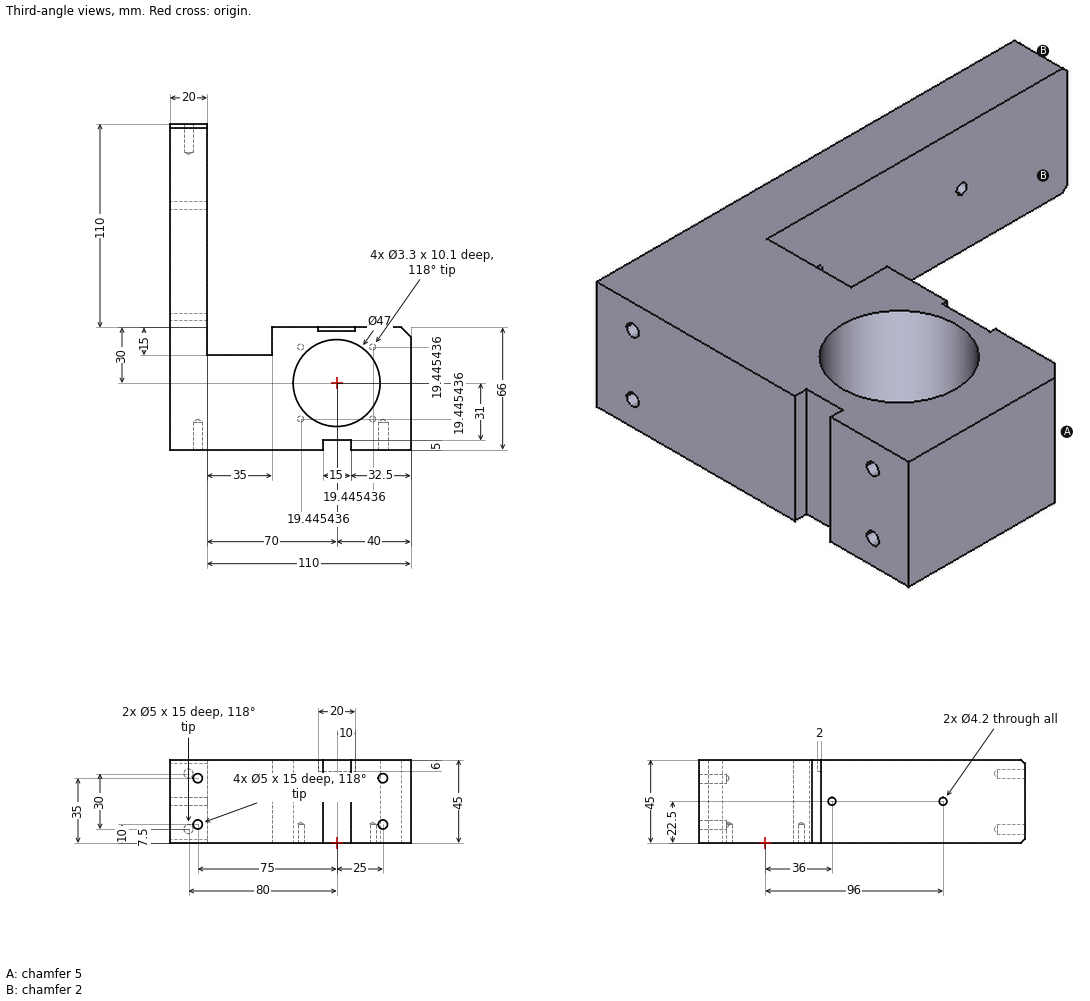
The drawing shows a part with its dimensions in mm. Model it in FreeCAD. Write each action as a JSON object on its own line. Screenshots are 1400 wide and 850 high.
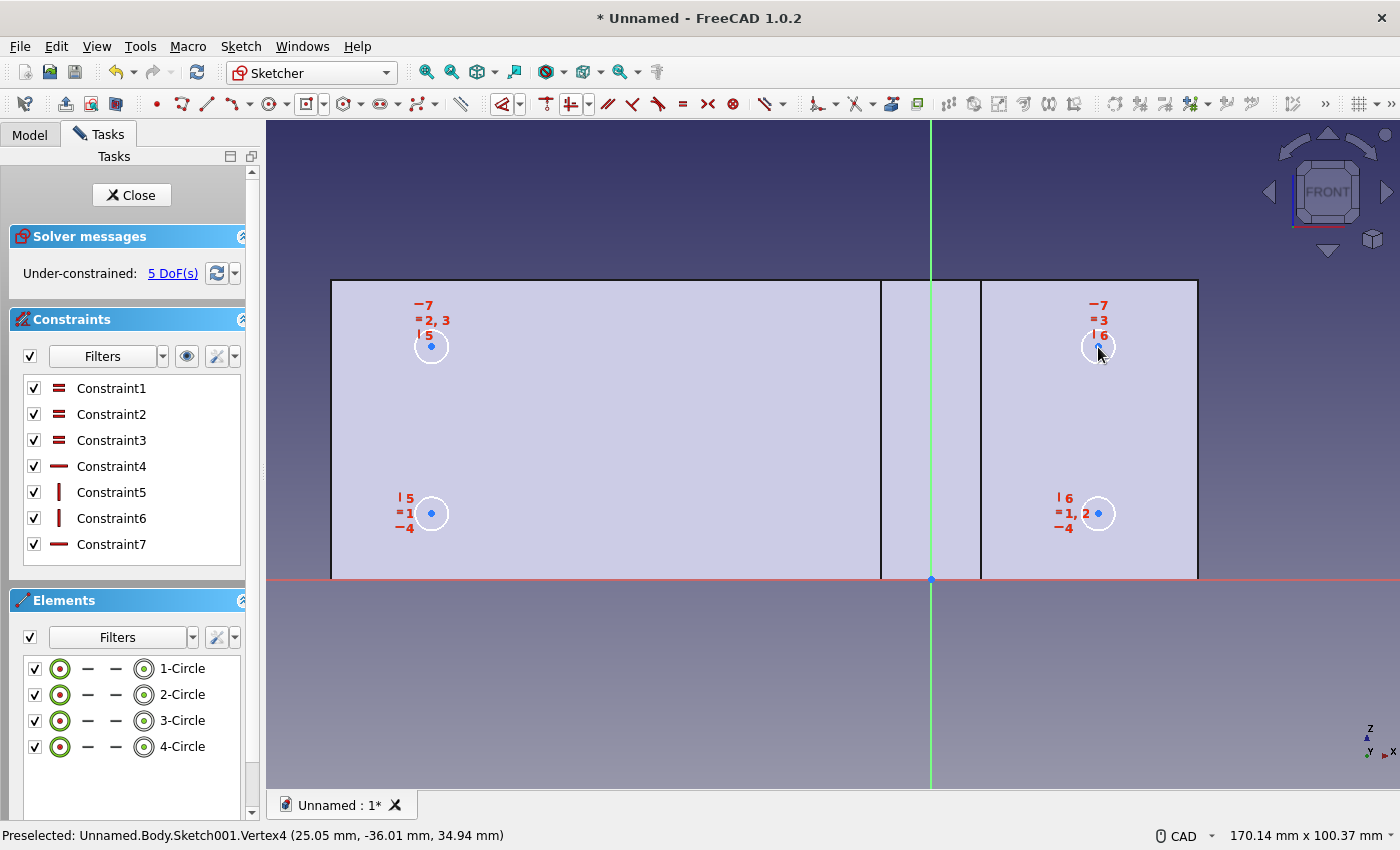
{"action": "left_click", "coordinate": [502, 104]}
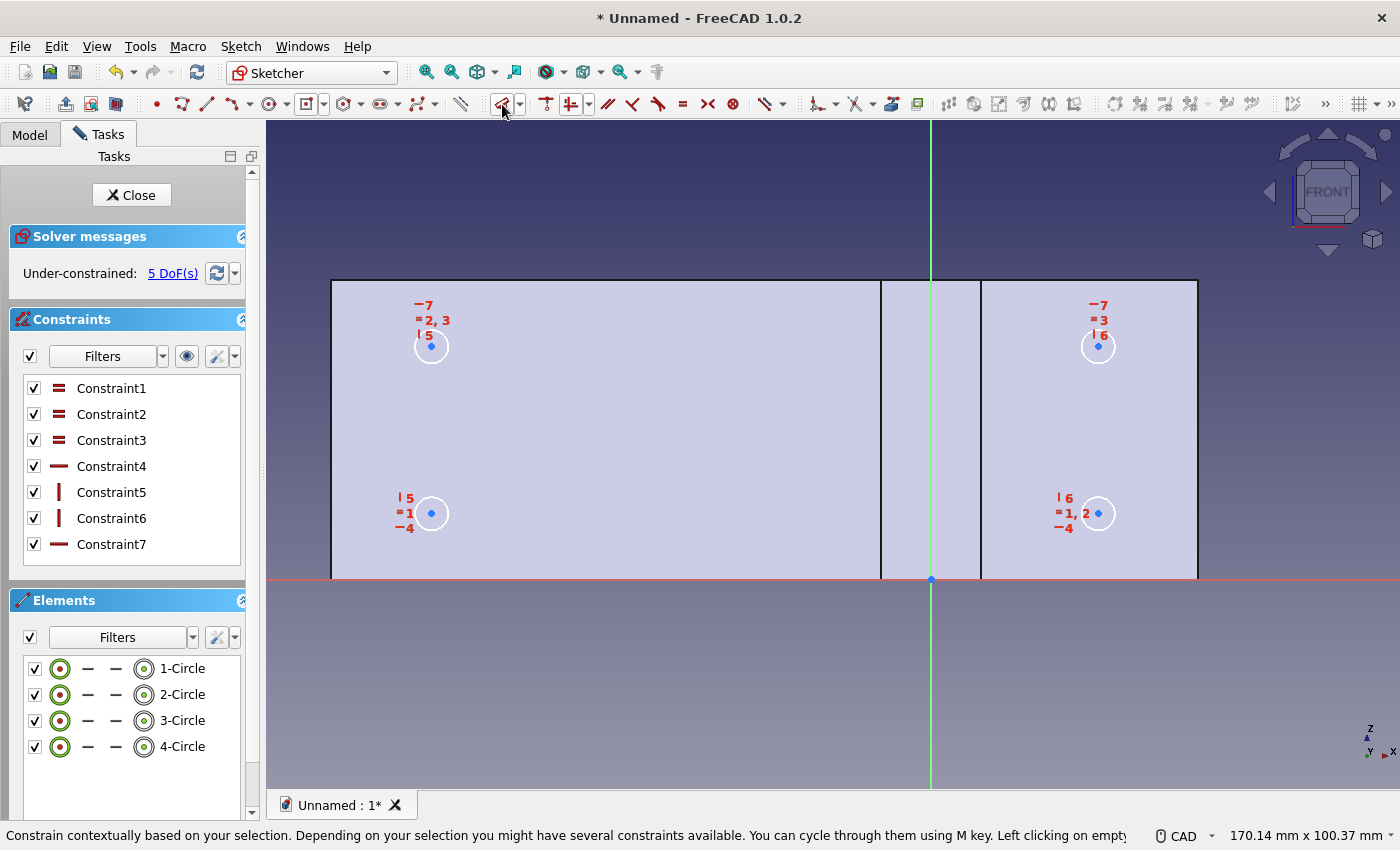
{"action": "left_click", "coordinate": [443, 502]}
{"action": "left_click", "coordinate": [465, 479]}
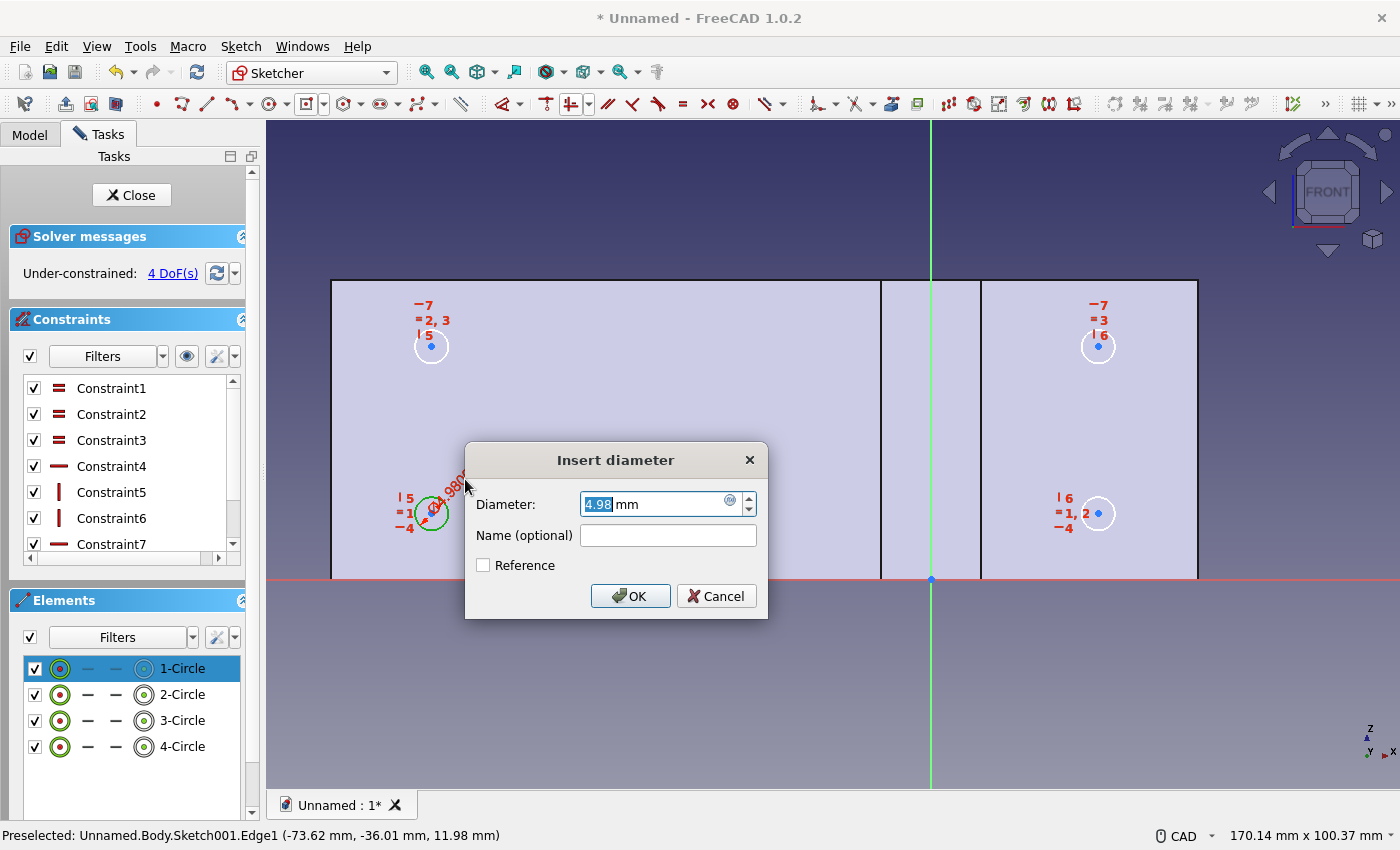
{"action": "type", "text": "5"}
{"action": "key", "text": "Return"}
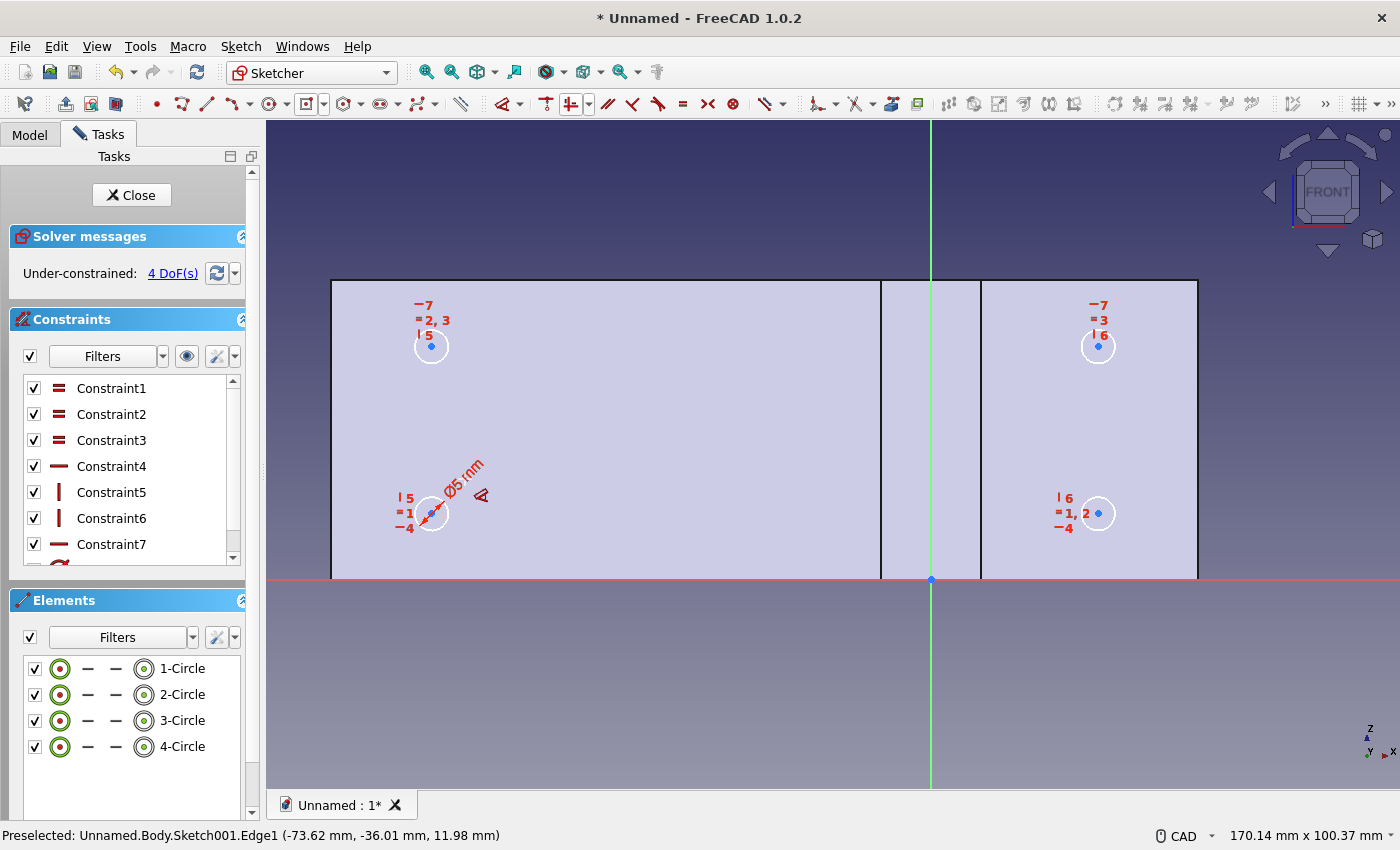
{"action": "left_click", "coordinate": [432, 514]}
{"action": "left_click", "coordinate": [682, 614]}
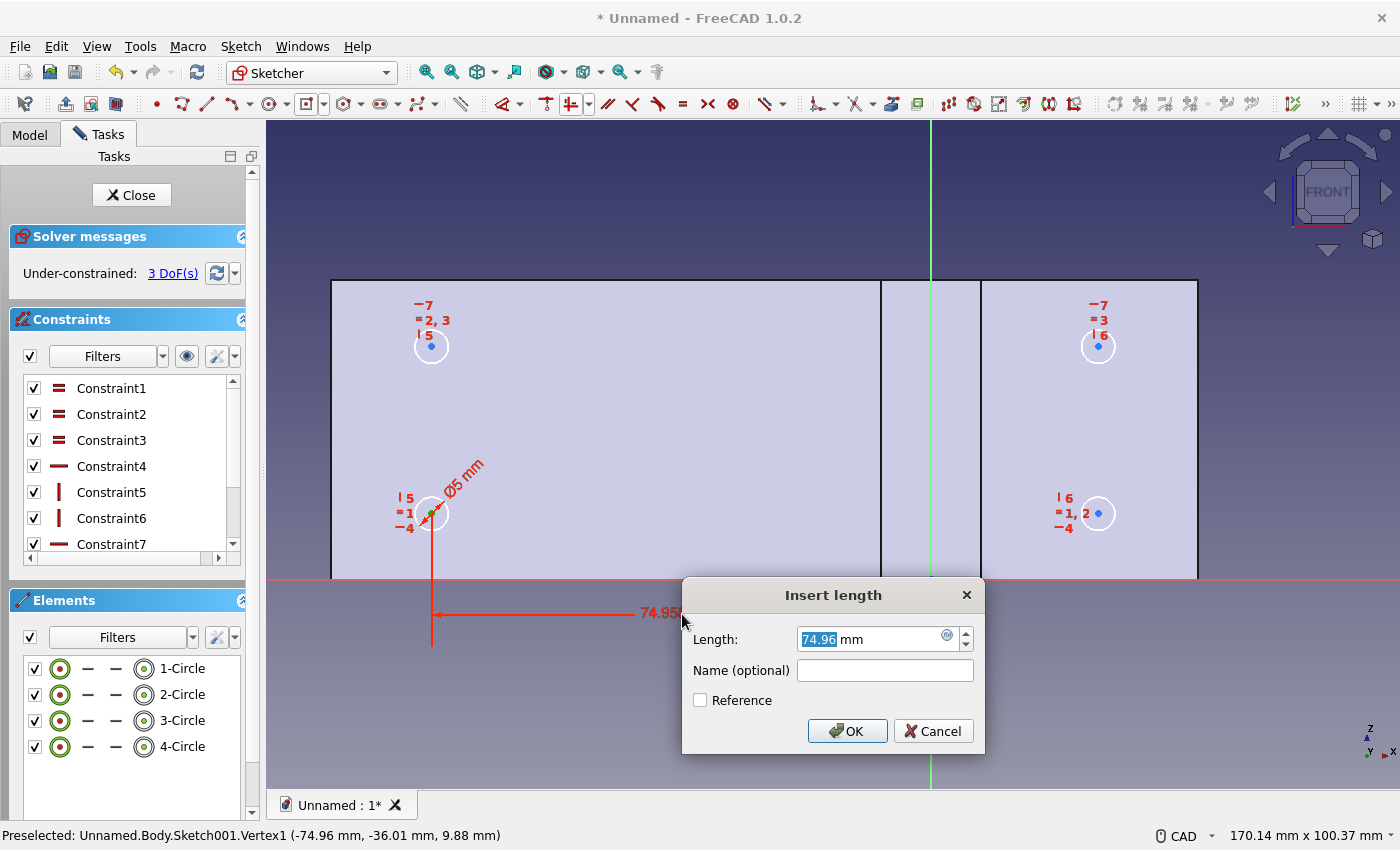
{"action": "type", "text": "75"}
{"action": "key", "text": "Return"}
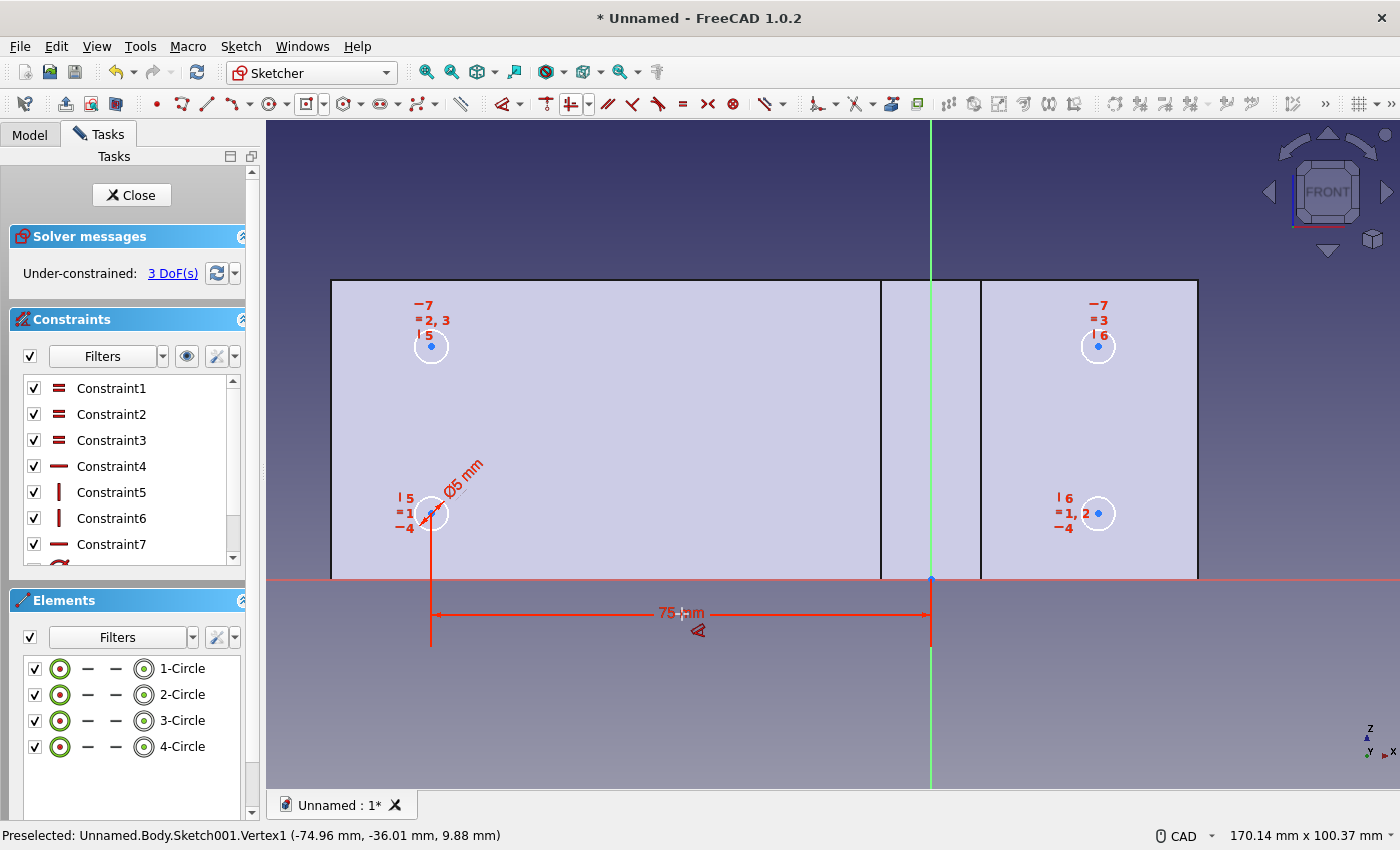
{"action": "left_click", "coordinate": [431, 514]}
{"action": "left_click", "coordinate": [397, 547]}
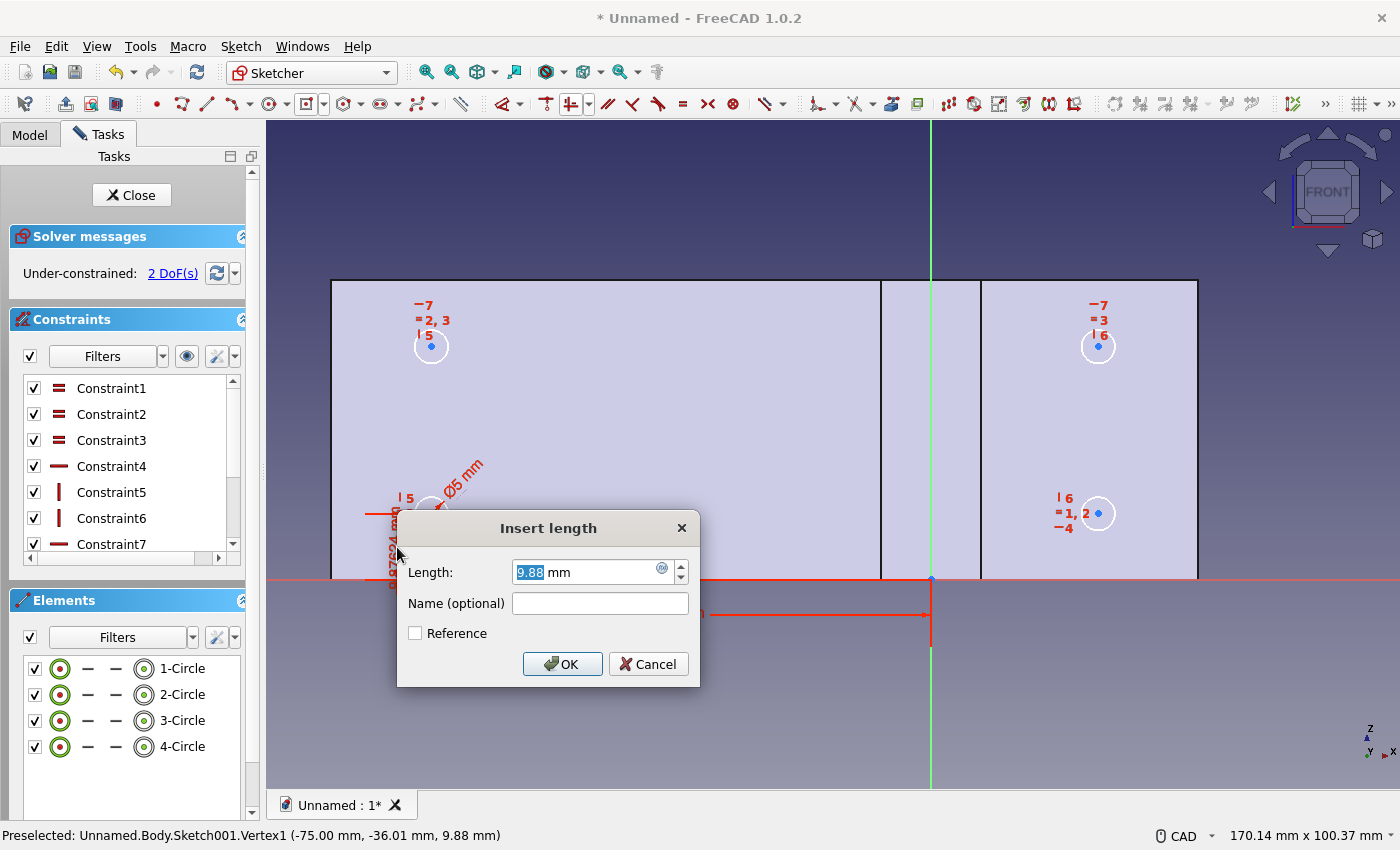
{"action": "type", "text": "10"}
{"action": "key", "text": "Return"}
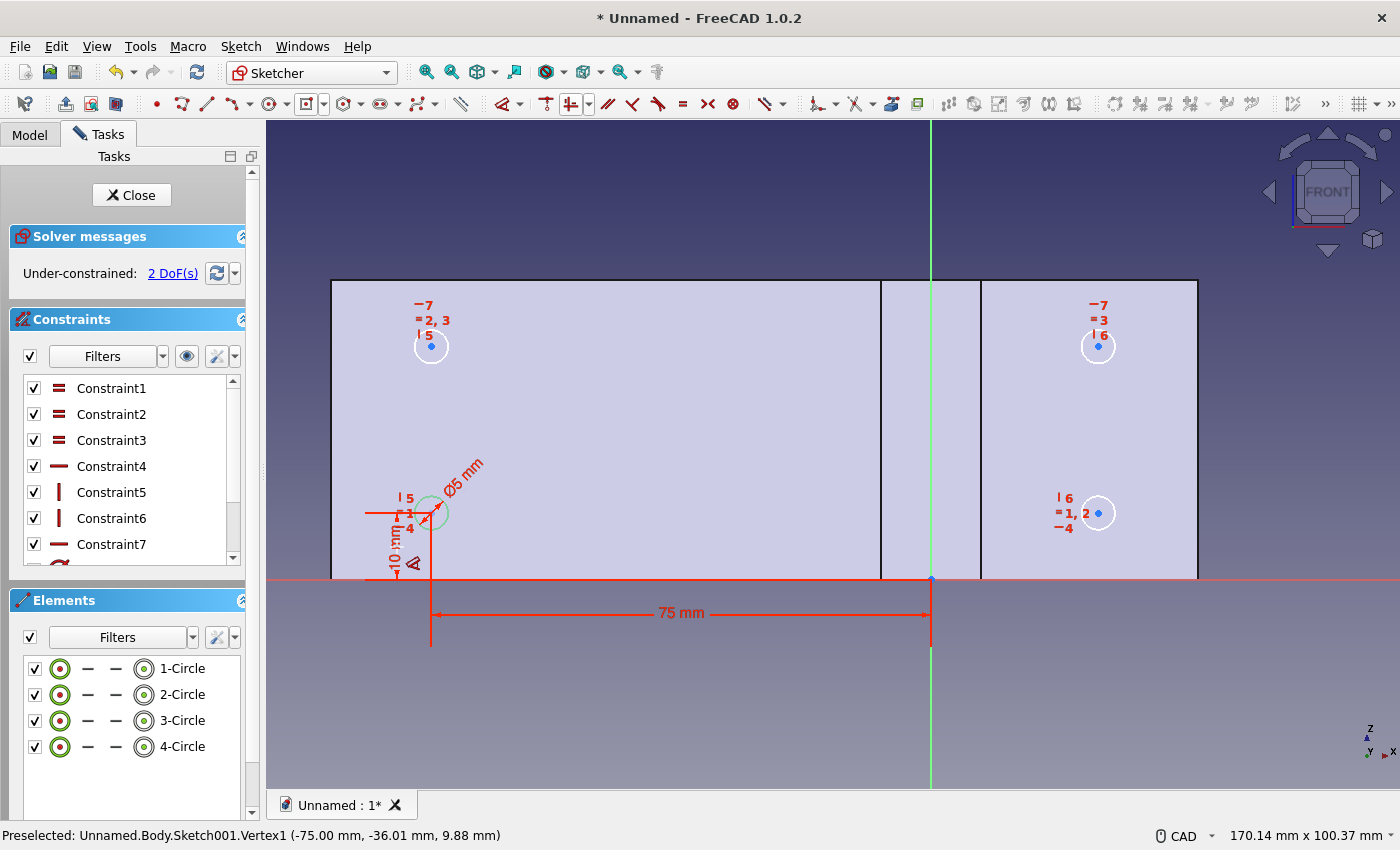
{"action": "left_click", "coordinate": [1098, 513]}
{"action": "left_click", "coordinate": [1015, 614]}